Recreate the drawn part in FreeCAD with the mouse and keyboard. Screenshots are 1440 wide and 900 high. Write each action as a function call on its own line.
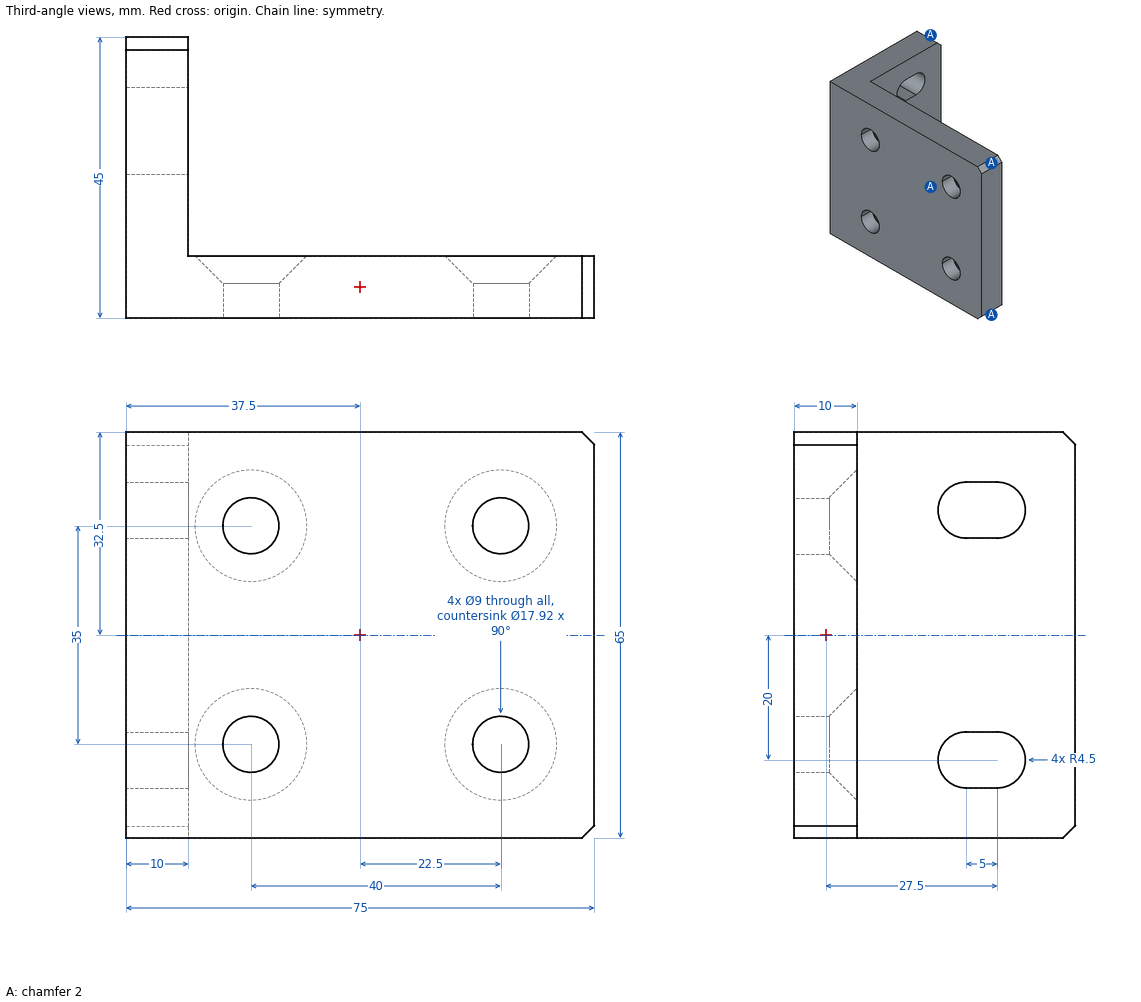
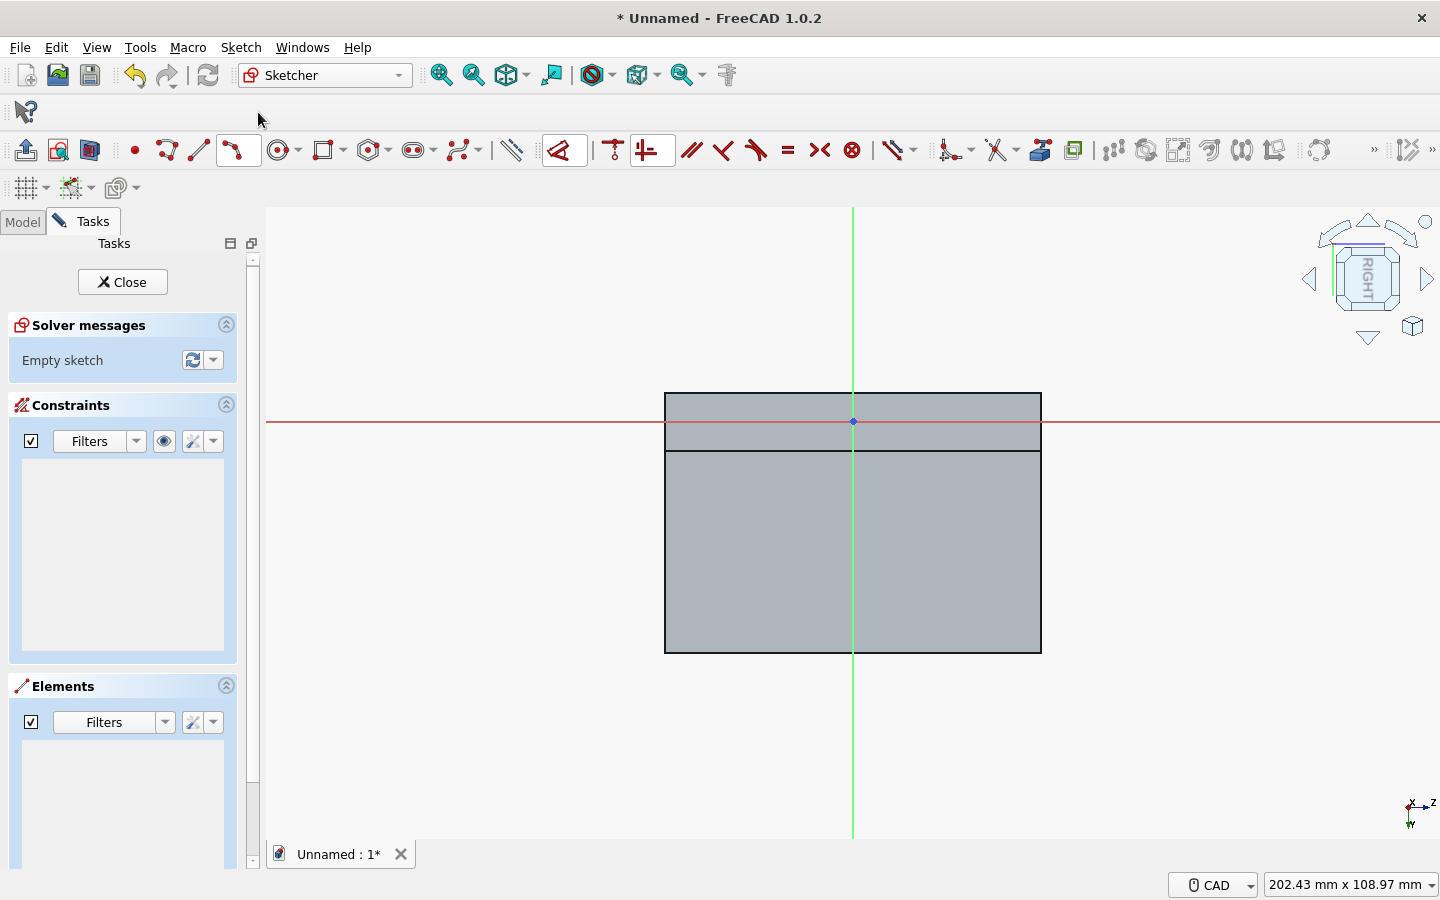
scroll(909, 507, up, 4)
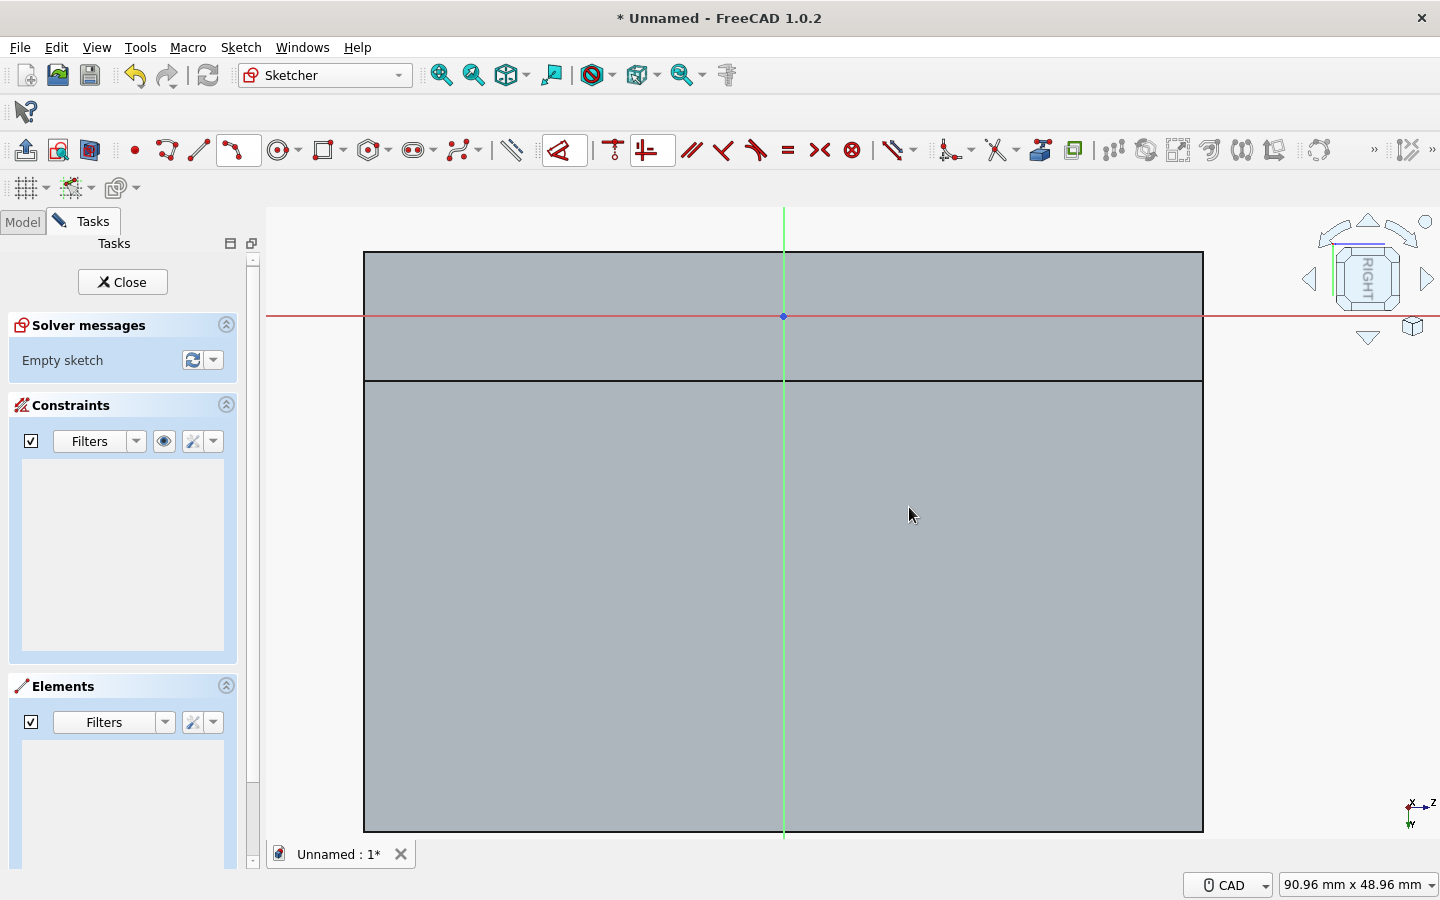
key(g)
key(s)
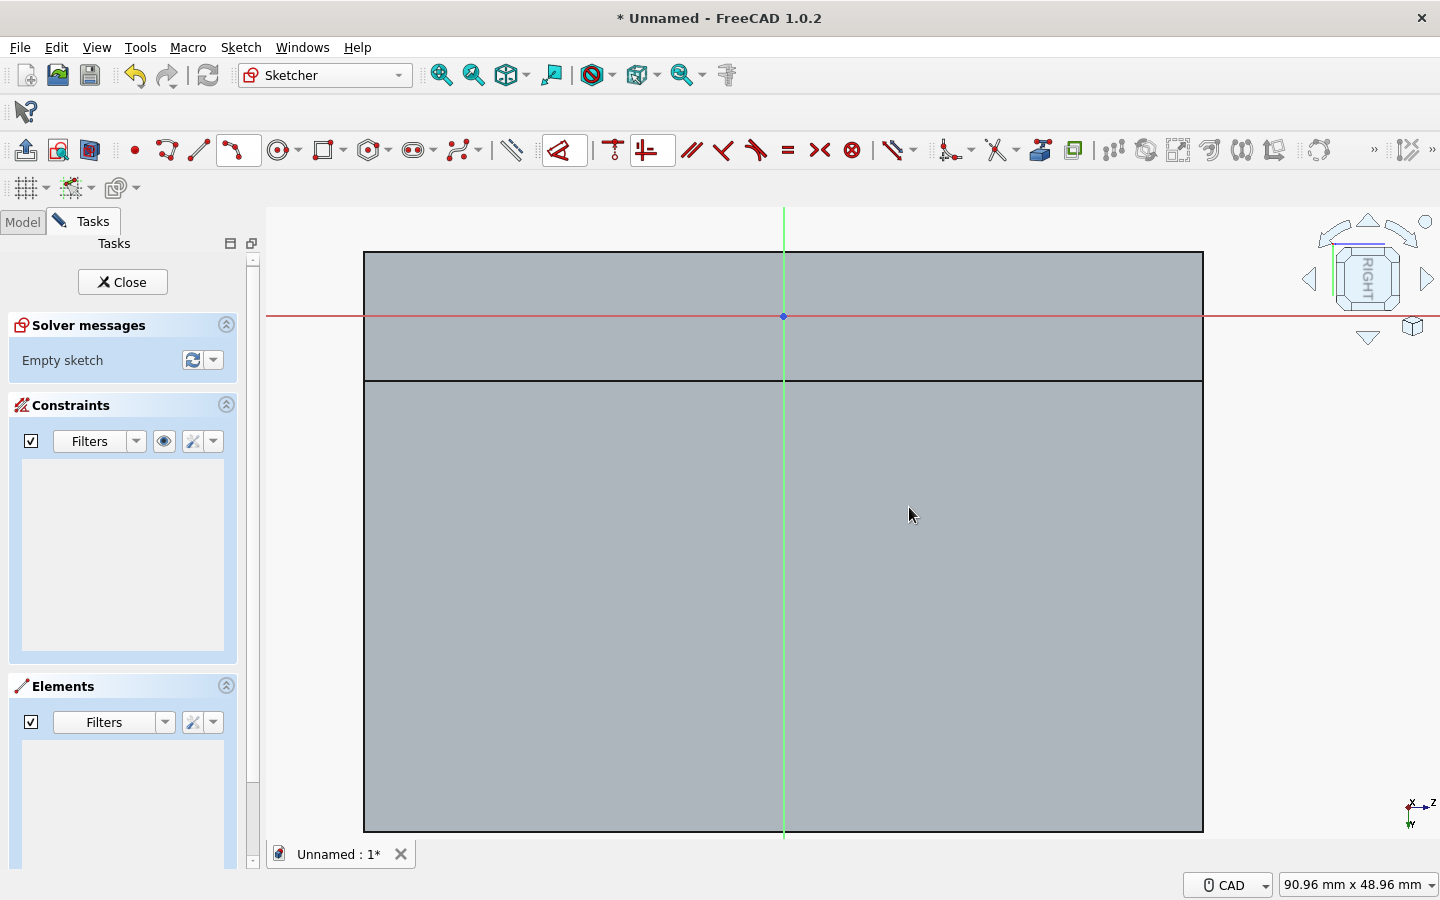
click(526, 671)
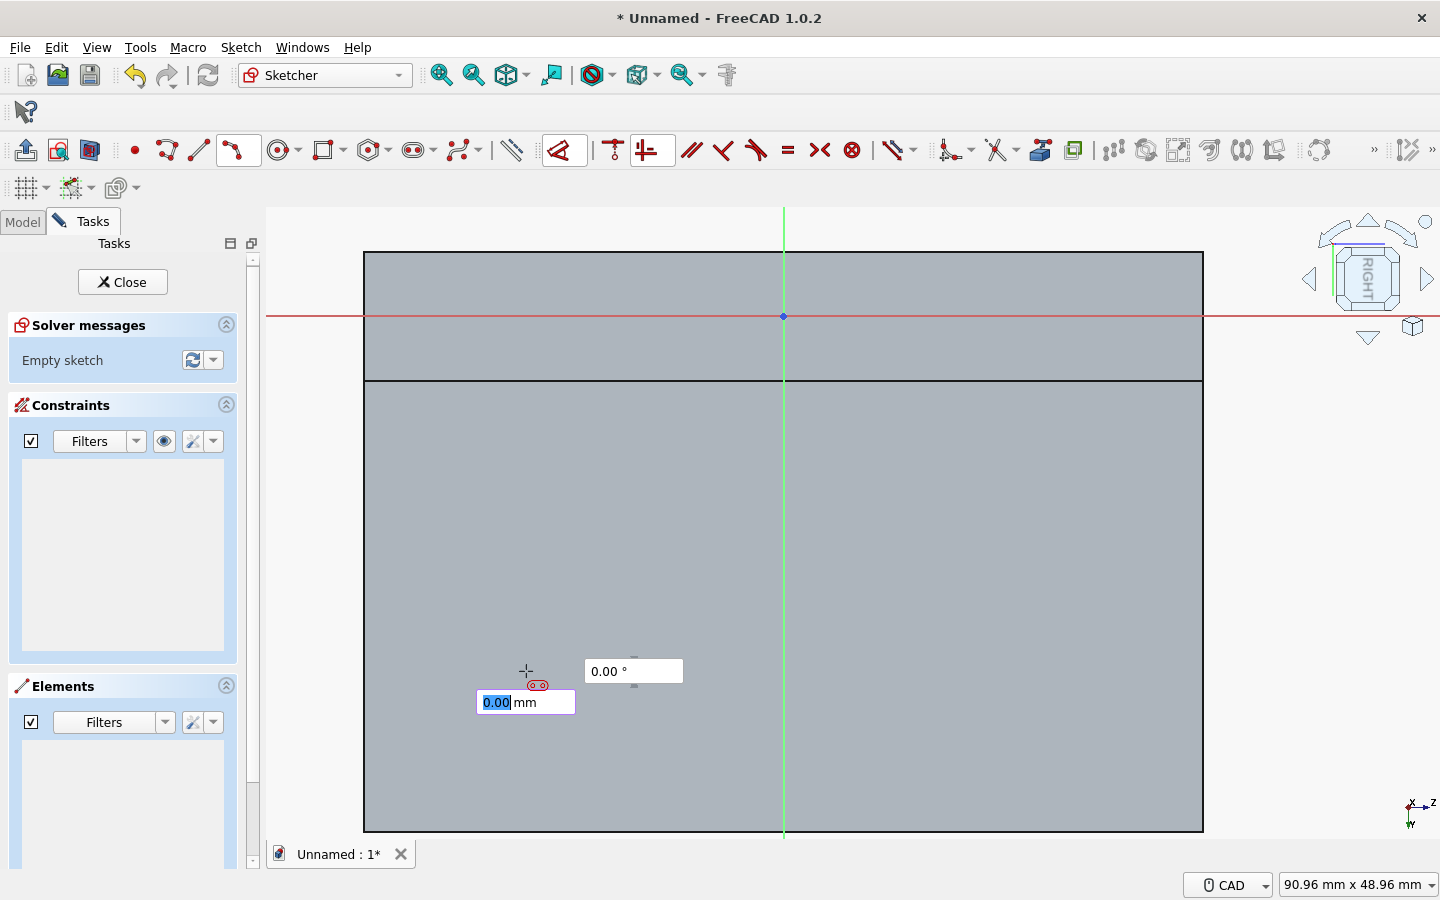
click(526, 607)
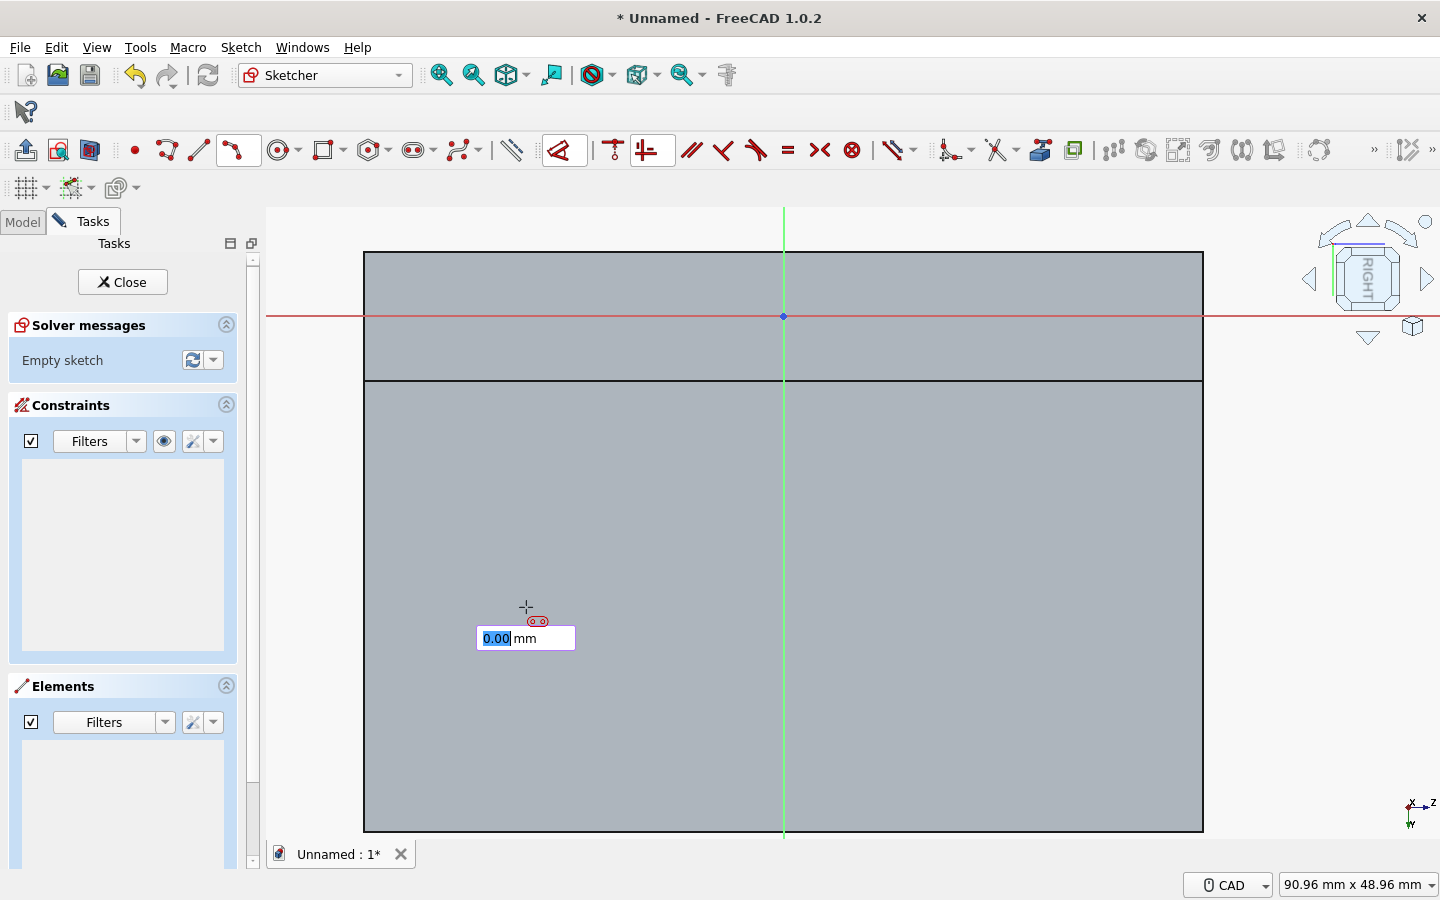
click(467, 639)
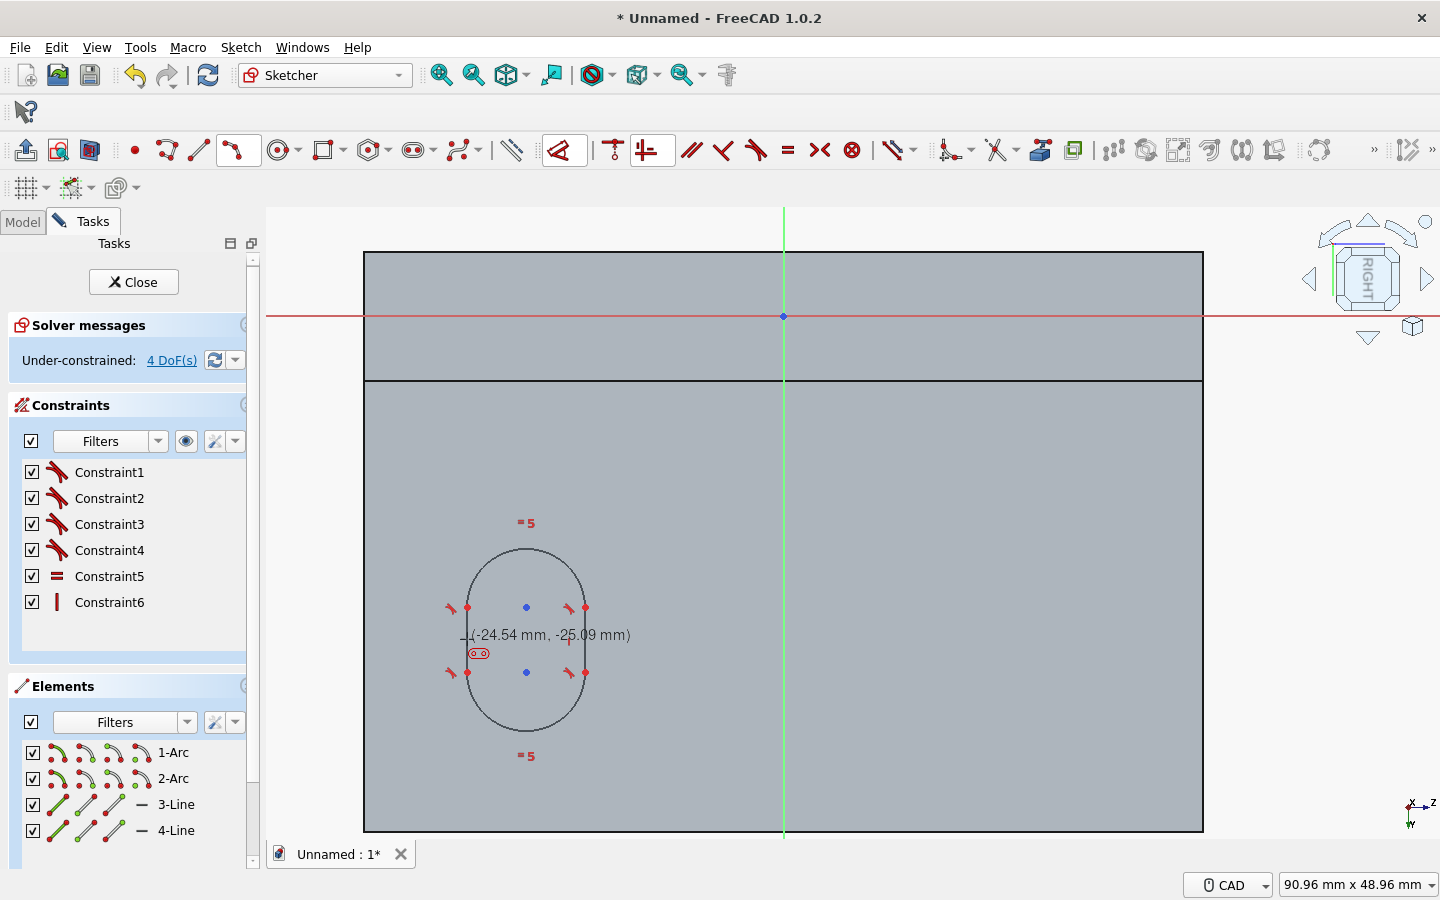
click(1042, 671)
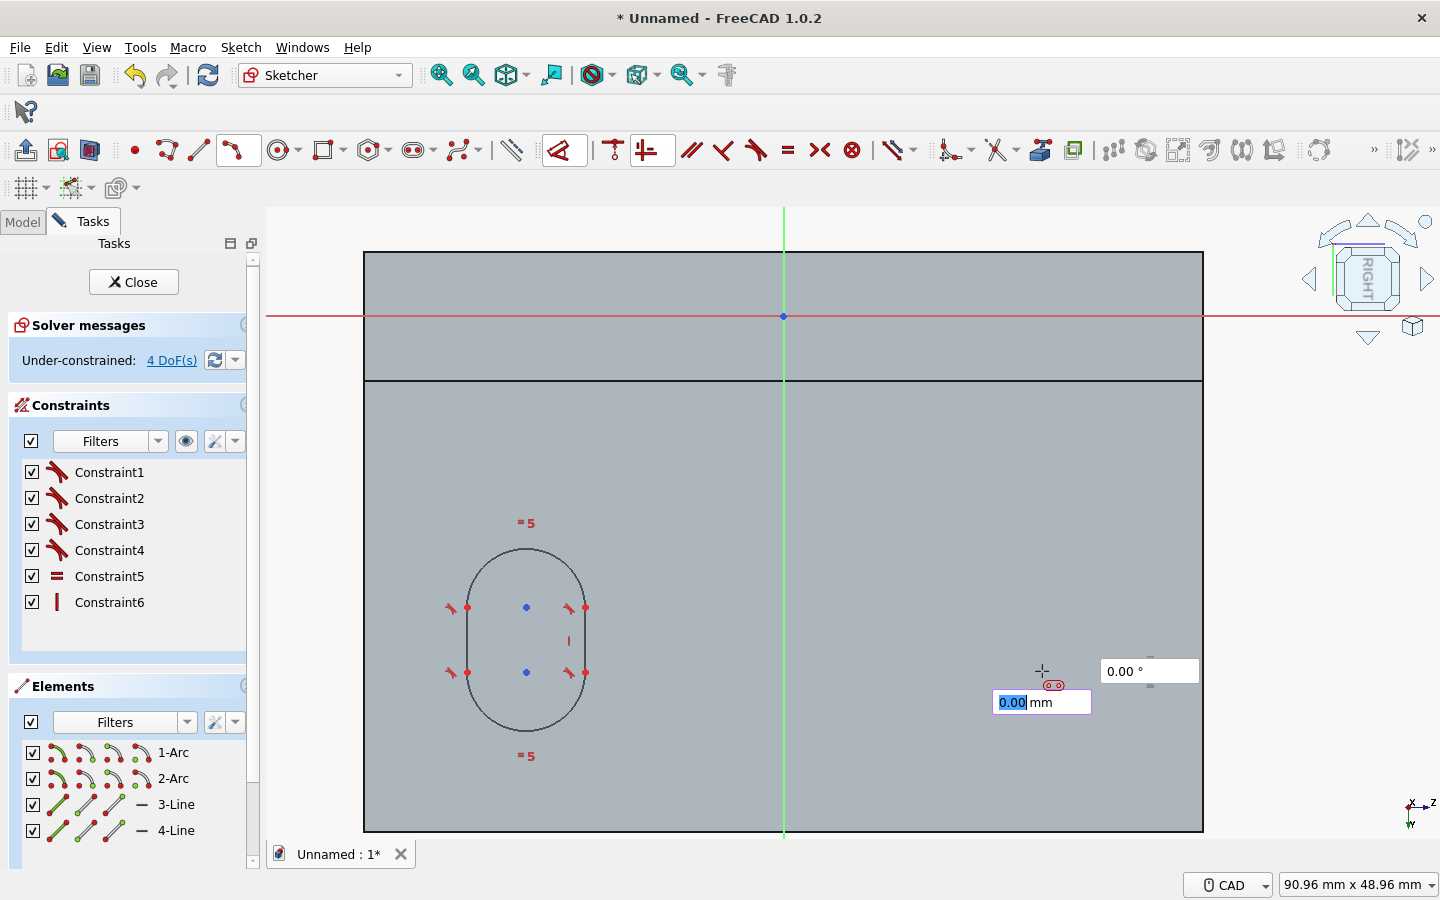
click(1042, 607)